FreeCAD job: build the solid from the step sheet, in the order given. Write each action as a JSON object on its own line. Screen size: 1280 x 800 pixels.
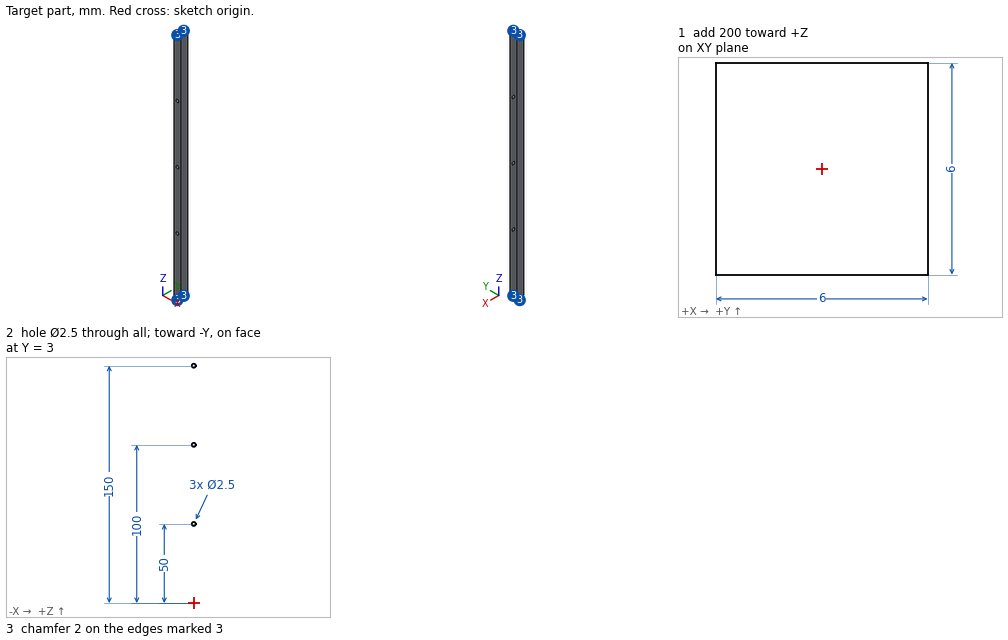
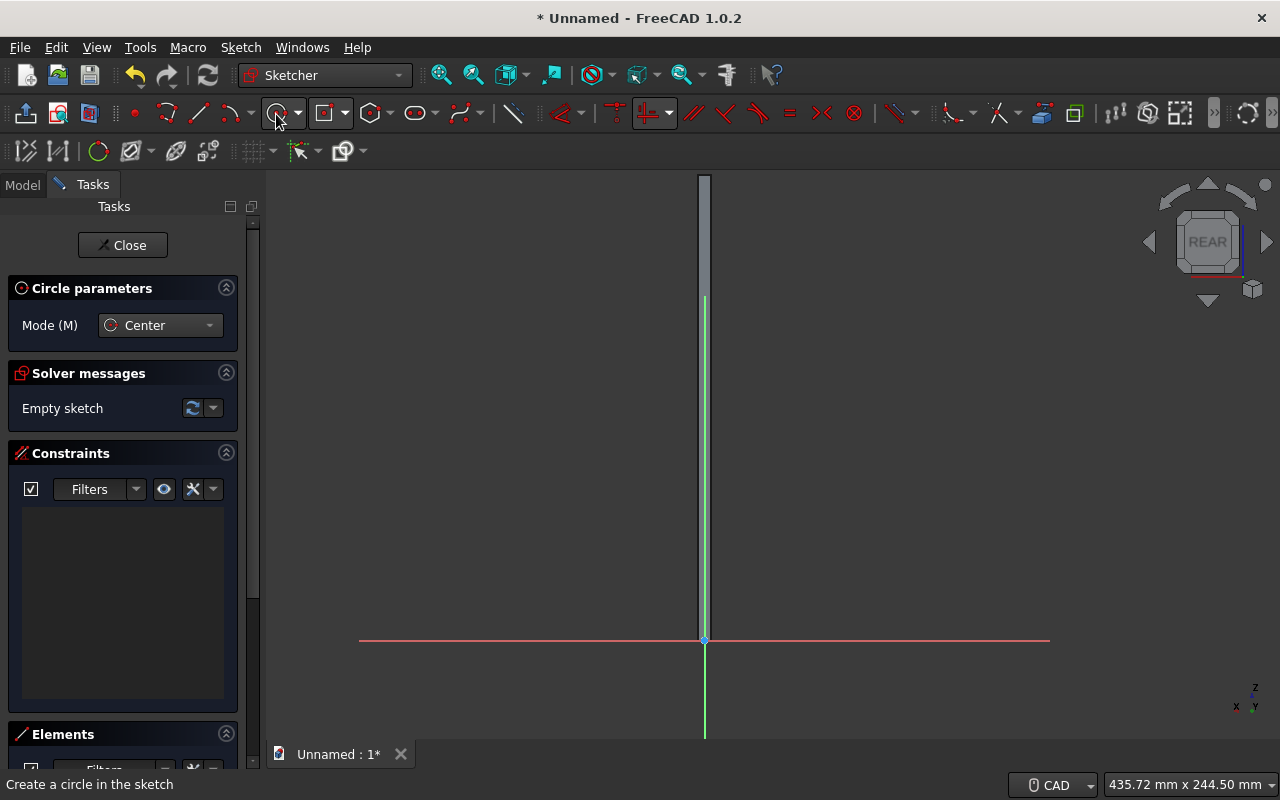
{"action": "scroll", "coordinate": [705, 524], "scroll_direction": "up", "scroll_amount": 11}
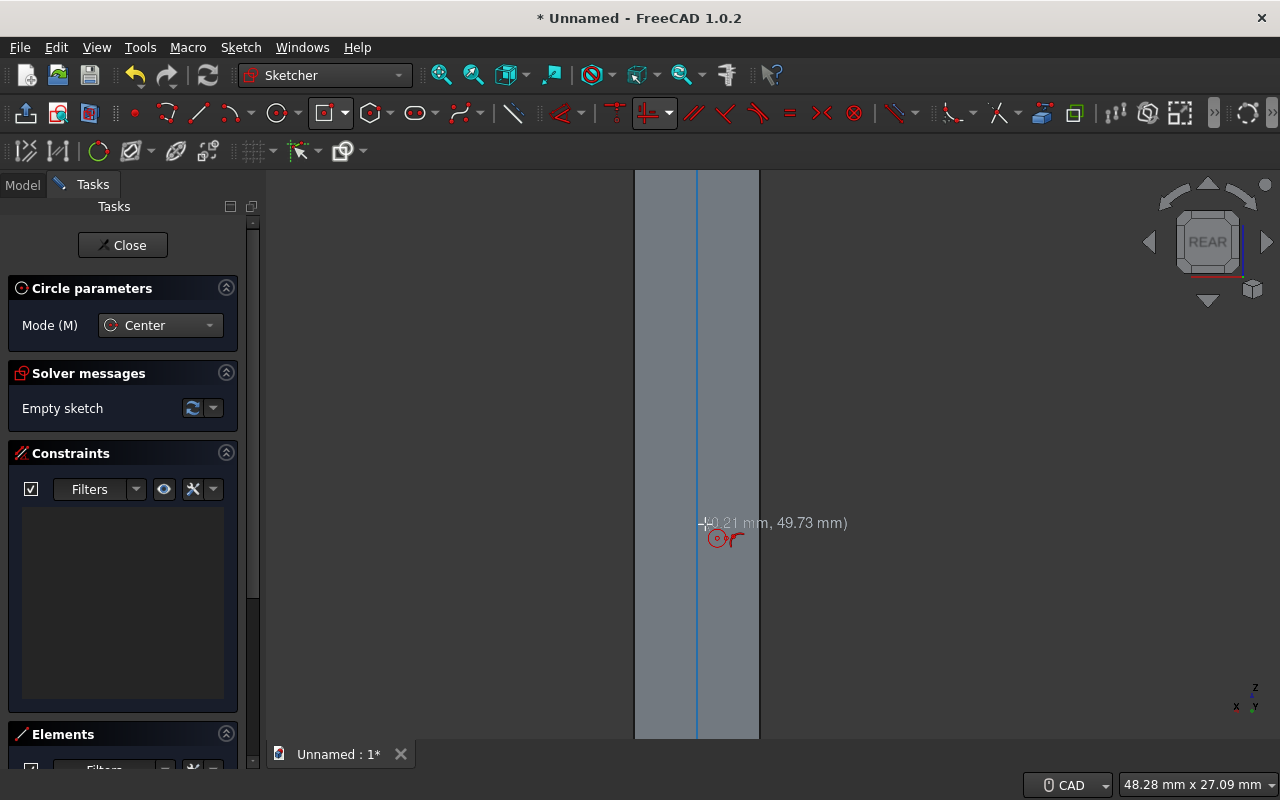
{"action": "scroll", "coordinate": [705, 513], "scroll_direction": "down", "scroll_amount": 11}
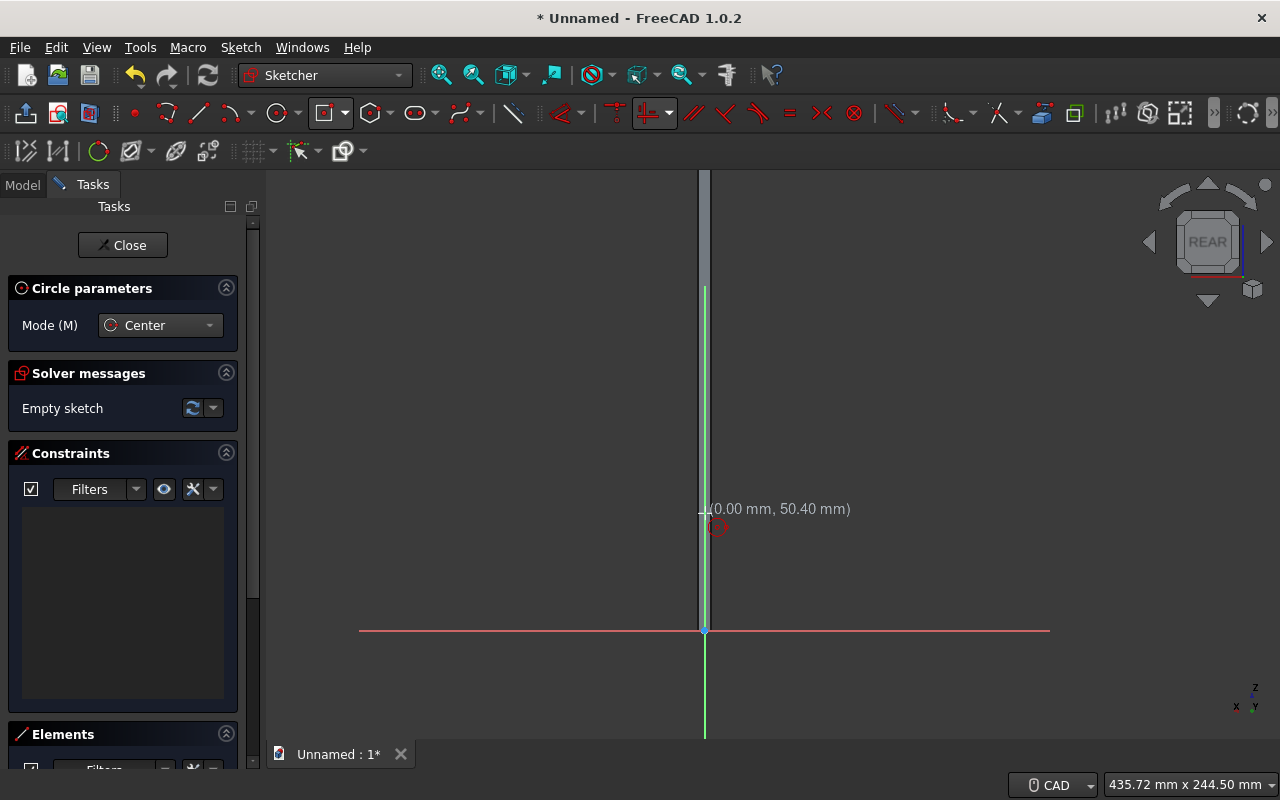
{"action": "left_click", "coordinate": [705, 515]}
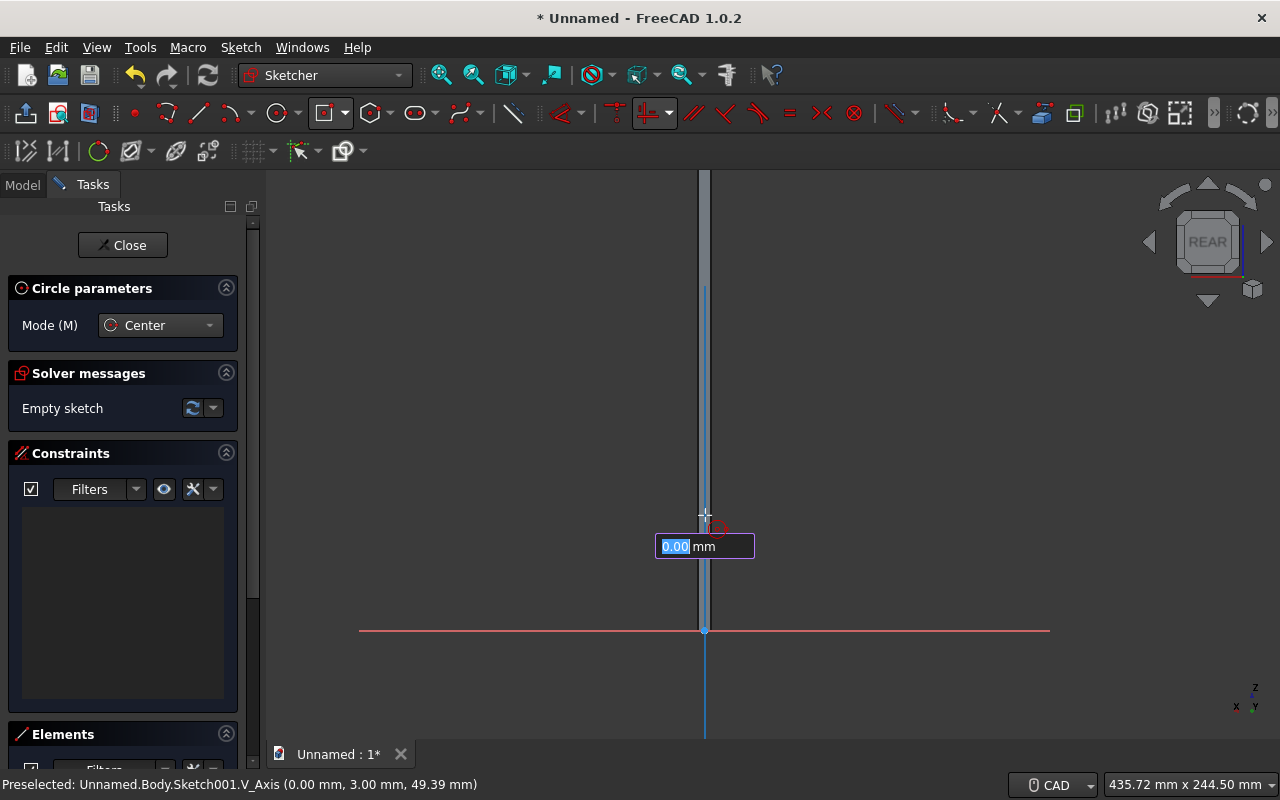
{"action": "scroll", "coordinate": [707, 514], "scroll_direction": "up", "scroll_amount": 9}
{"action": "mouse_move", "coordinate": [706, 508]}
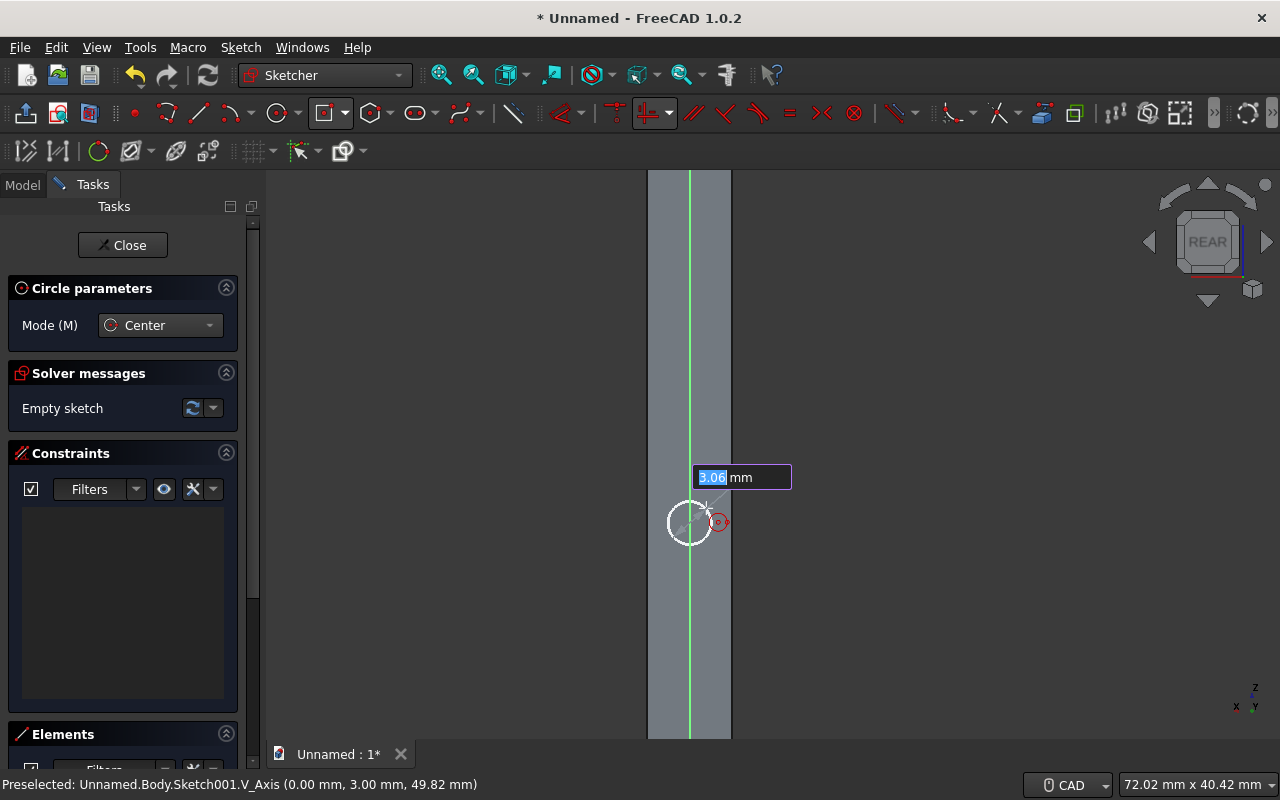
{"action": "type", "text": "2.5"}
{"action": "key", "text": "Return"}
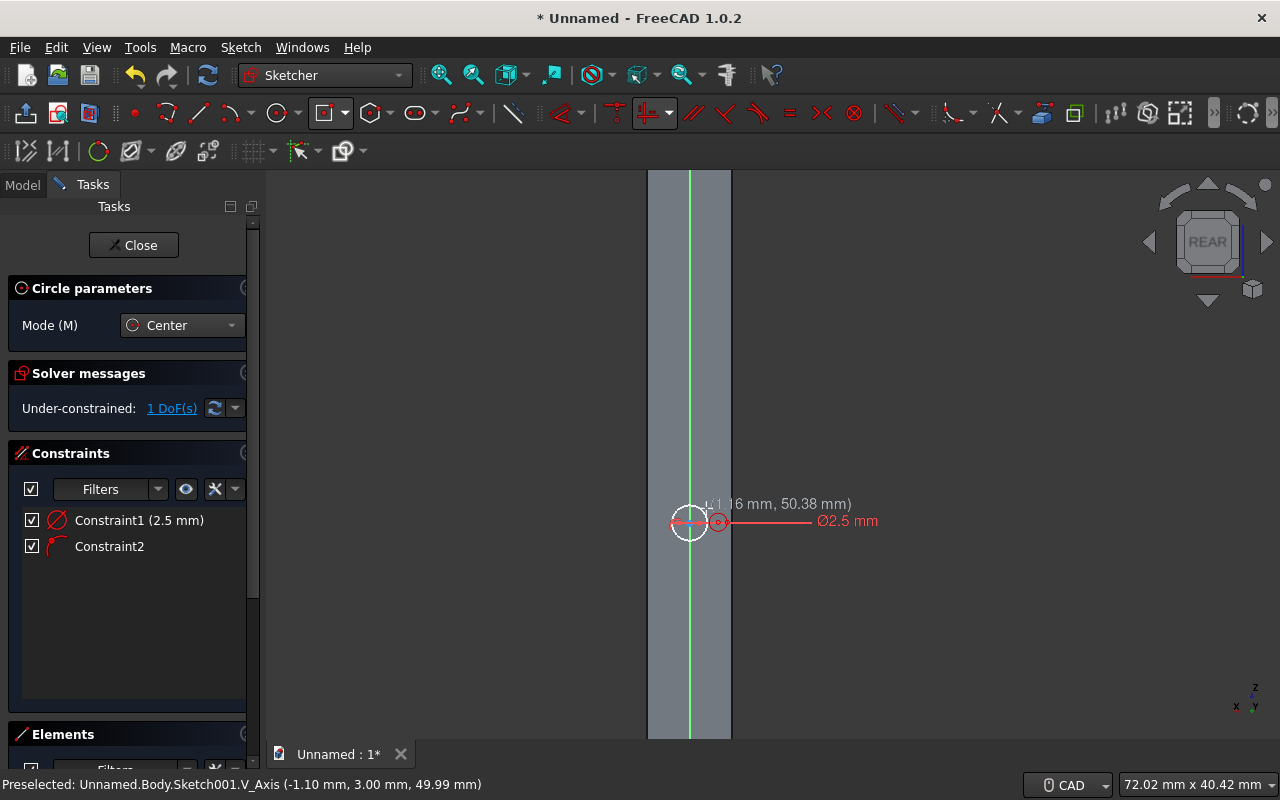
{"action": "scroll", "coordinate": [707, 514], "scroll_direction": "down", "scroll_amount": 9}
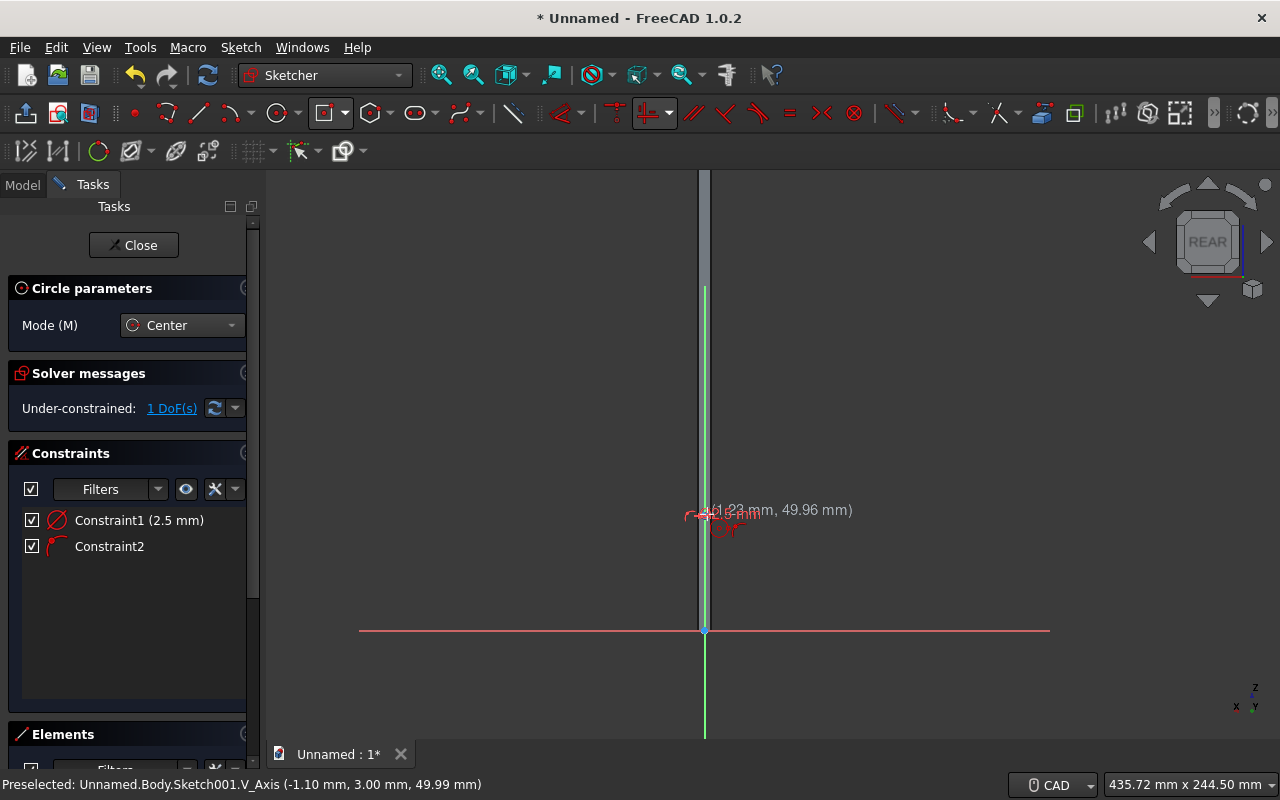
{"action": "scroll", "coordinate": [705, 398], "scroll_direction": "up", "scroll_amount": 11}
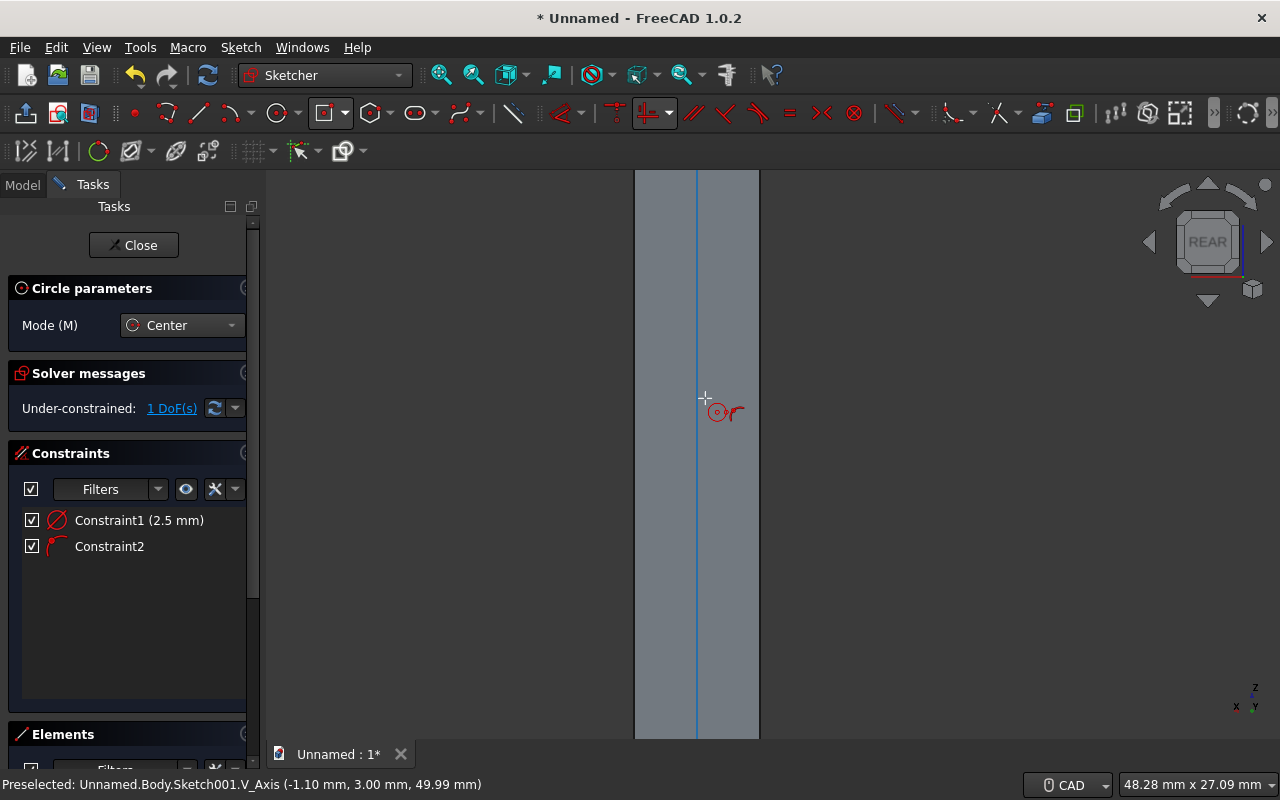
{"action": "scroll", "coordinate": [705, 398], "scroll_direction": "down", "scroll_amount": 11}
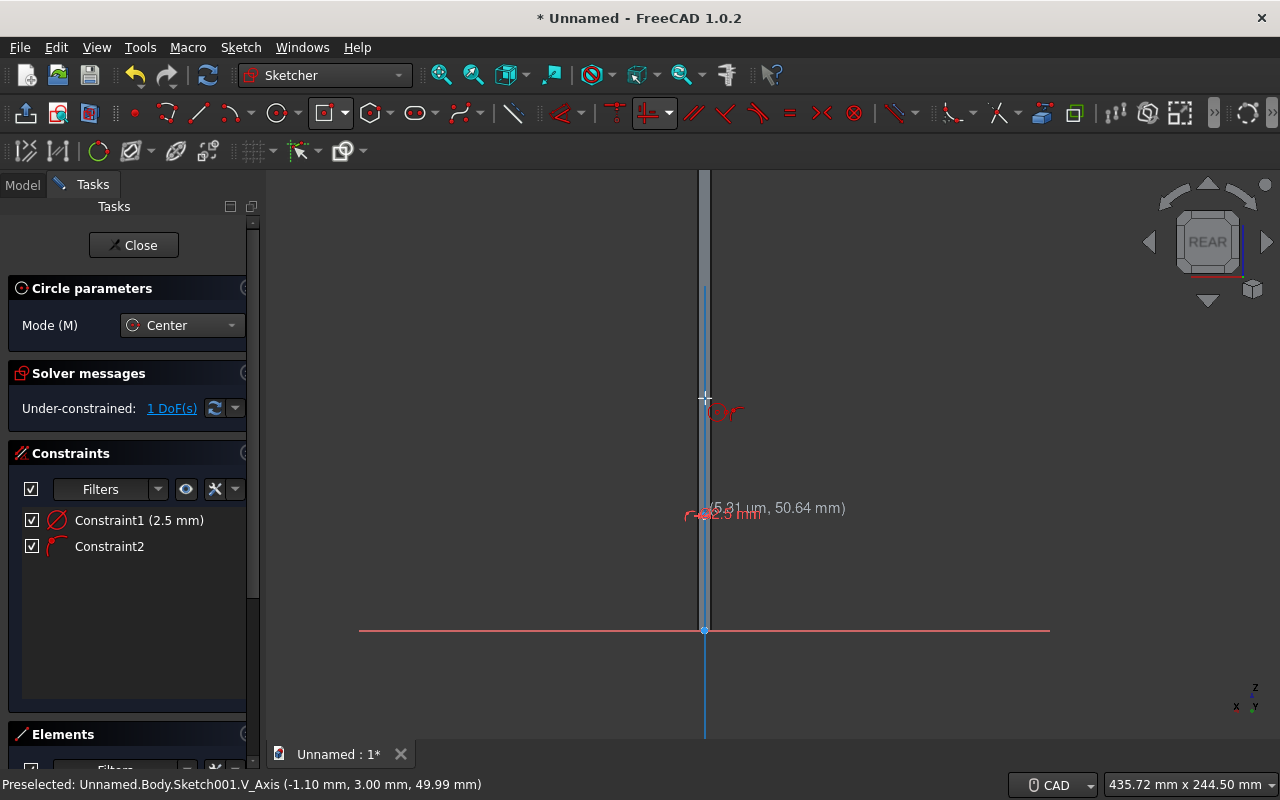
{"action": "left_click", "coordinate": [705, 398]}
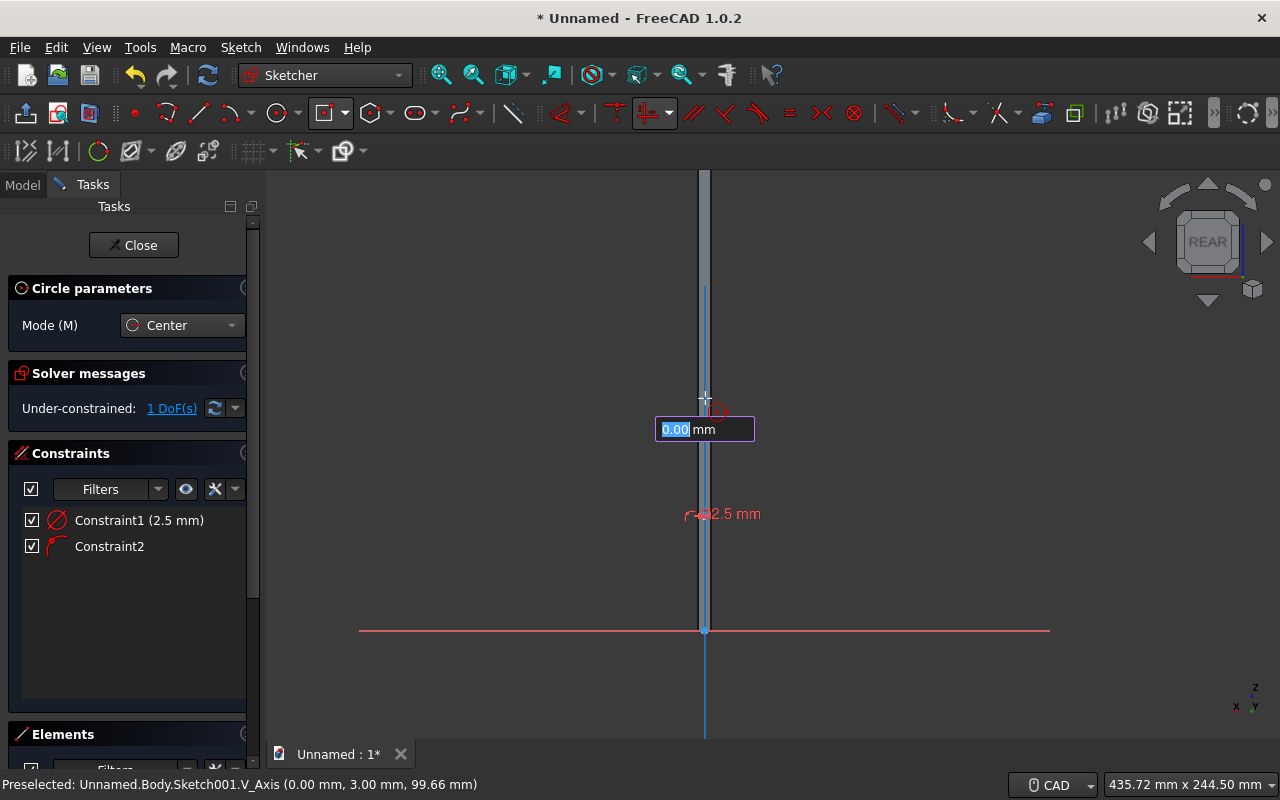
{"action": "scroll", "coordinate": [707, 397], "scroll_direction": "up", "scroll_amount": 9}
{"action": "mouse_move", "coordinate": [706, 396]}